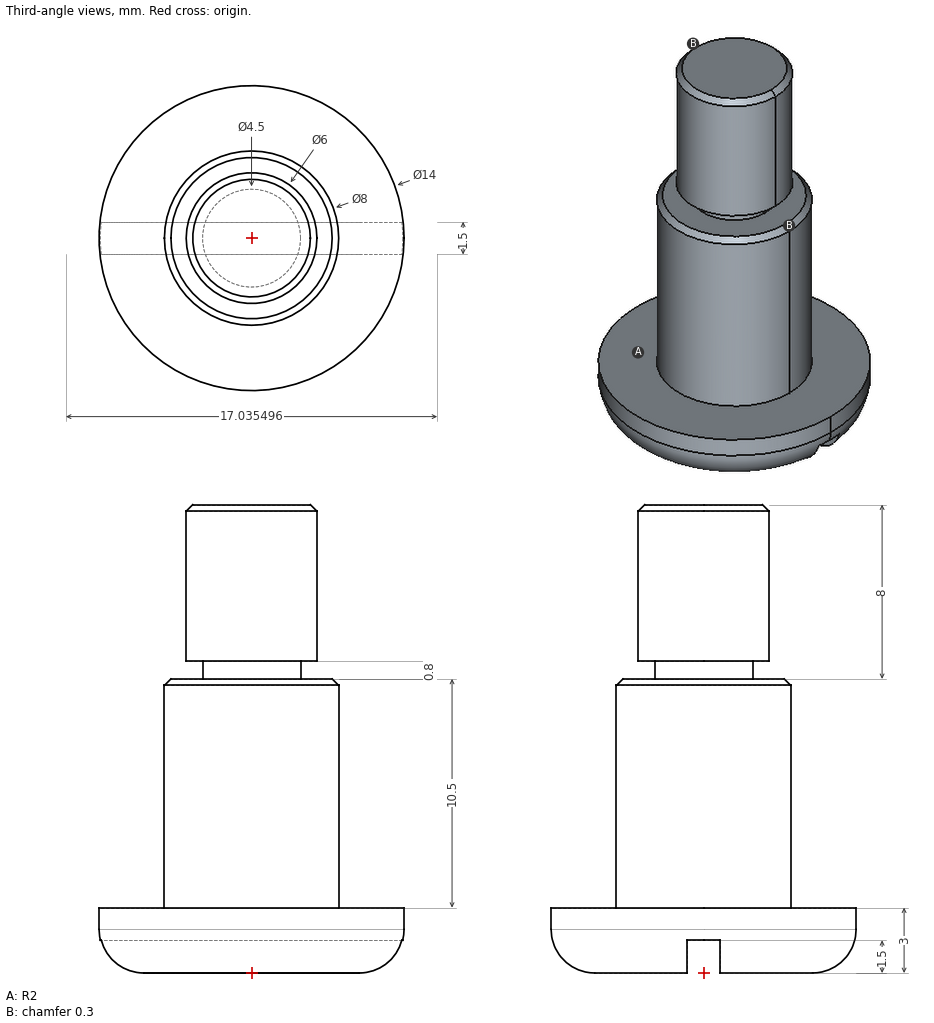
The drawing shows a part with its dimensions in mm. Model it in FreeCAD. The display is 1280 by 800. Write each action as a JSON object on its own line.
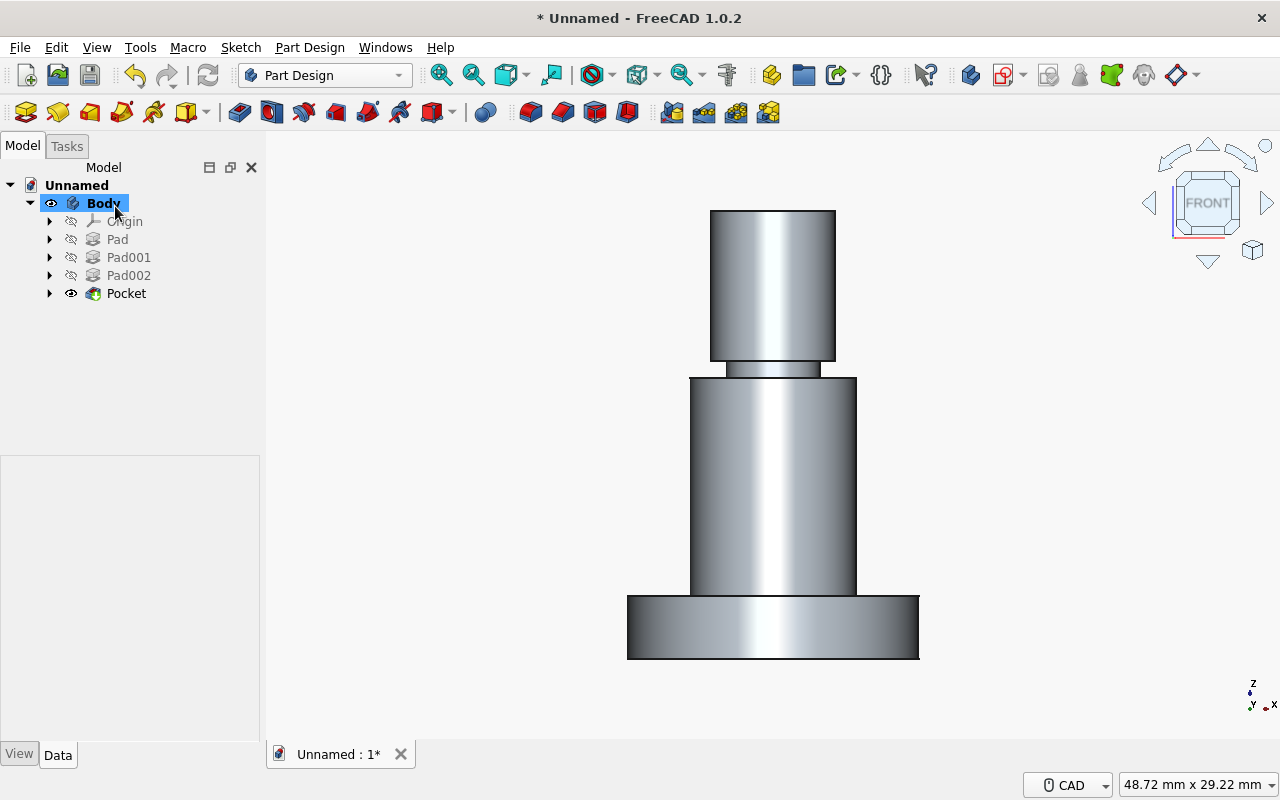
{"action": "left_click", "coordinate": [655, 658]}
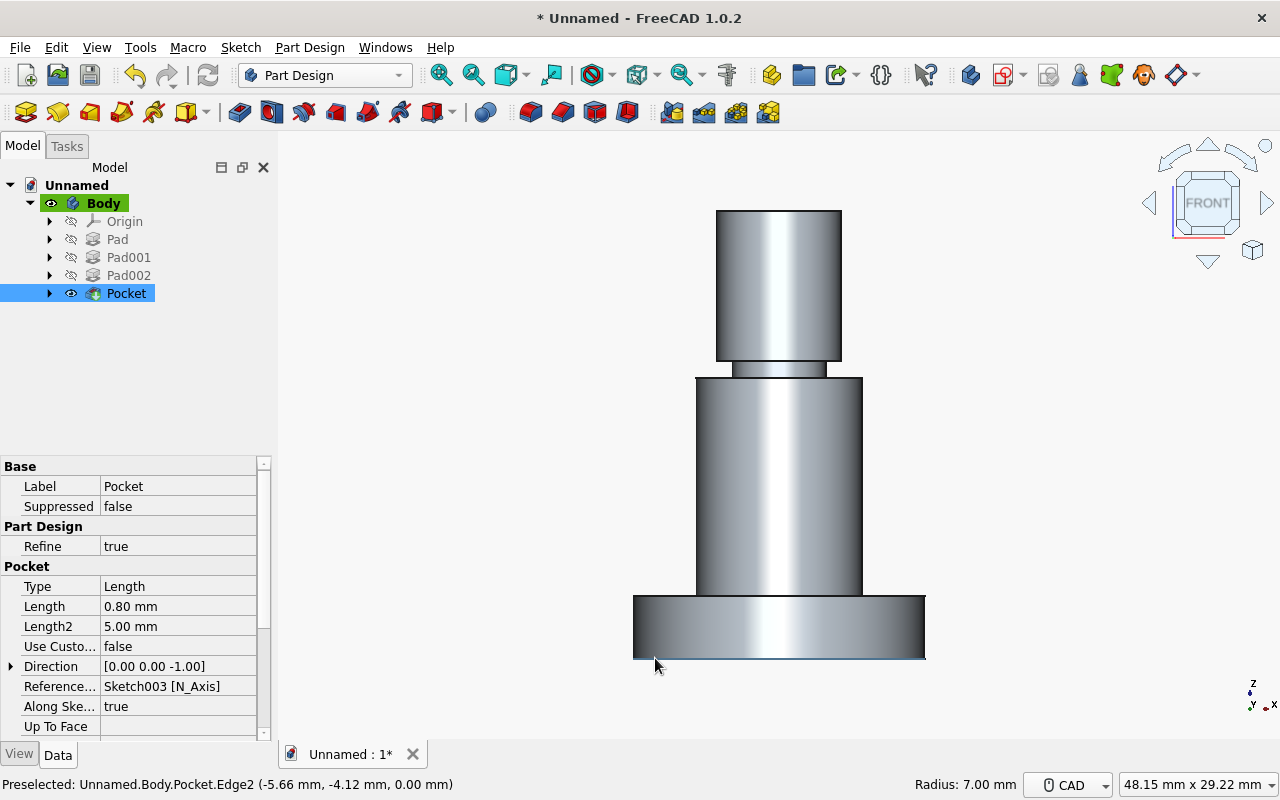
{"action": "left_click", "coordinate": [532, 112]}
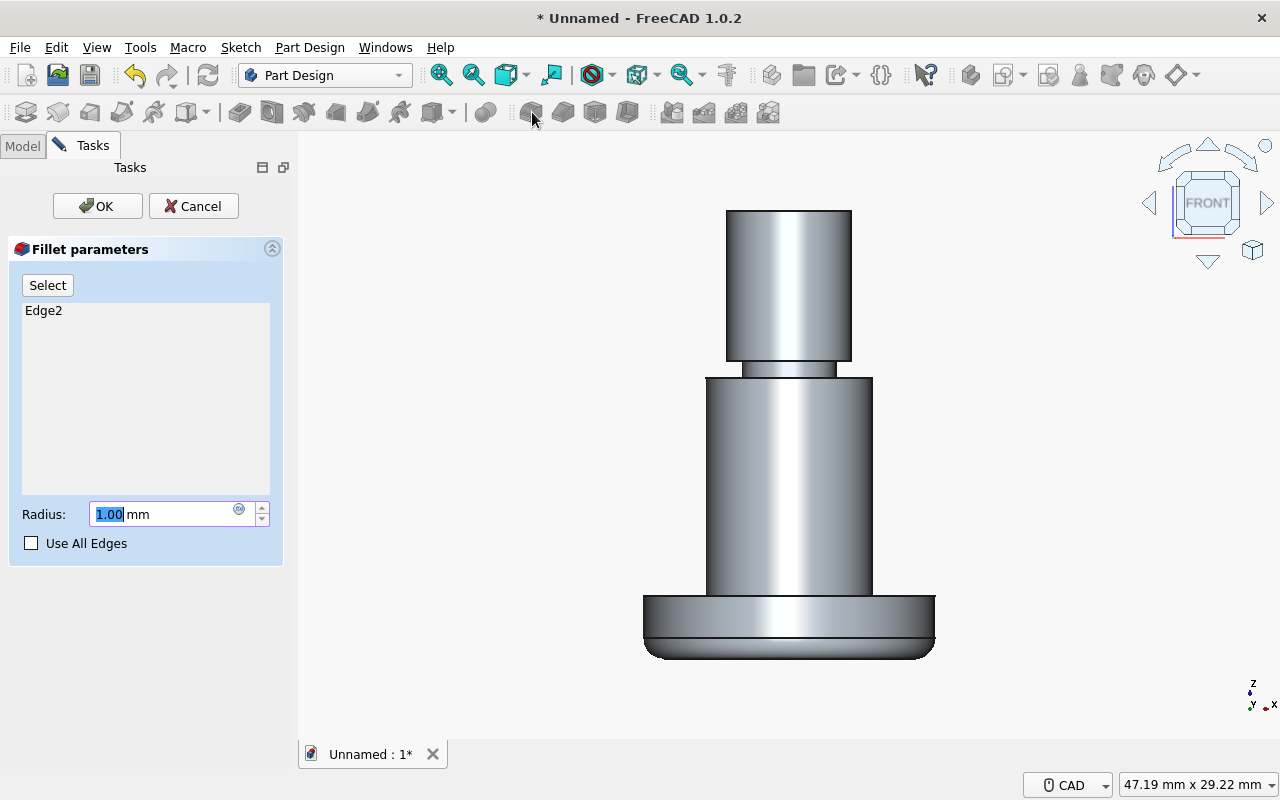
{"action": "type", "text": "2"}
{"action": "key", "text": "Tab"}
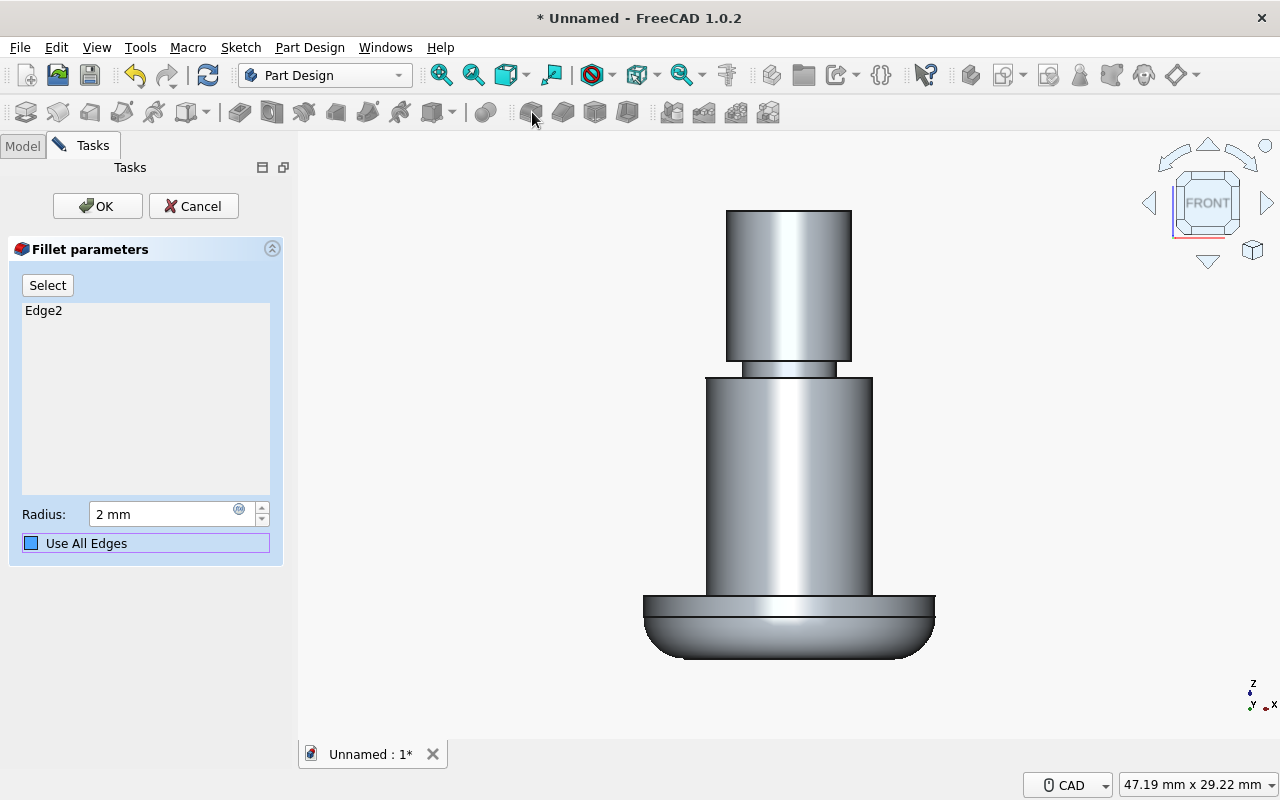
{"action": "left_click", "coordinate": [98, 206]}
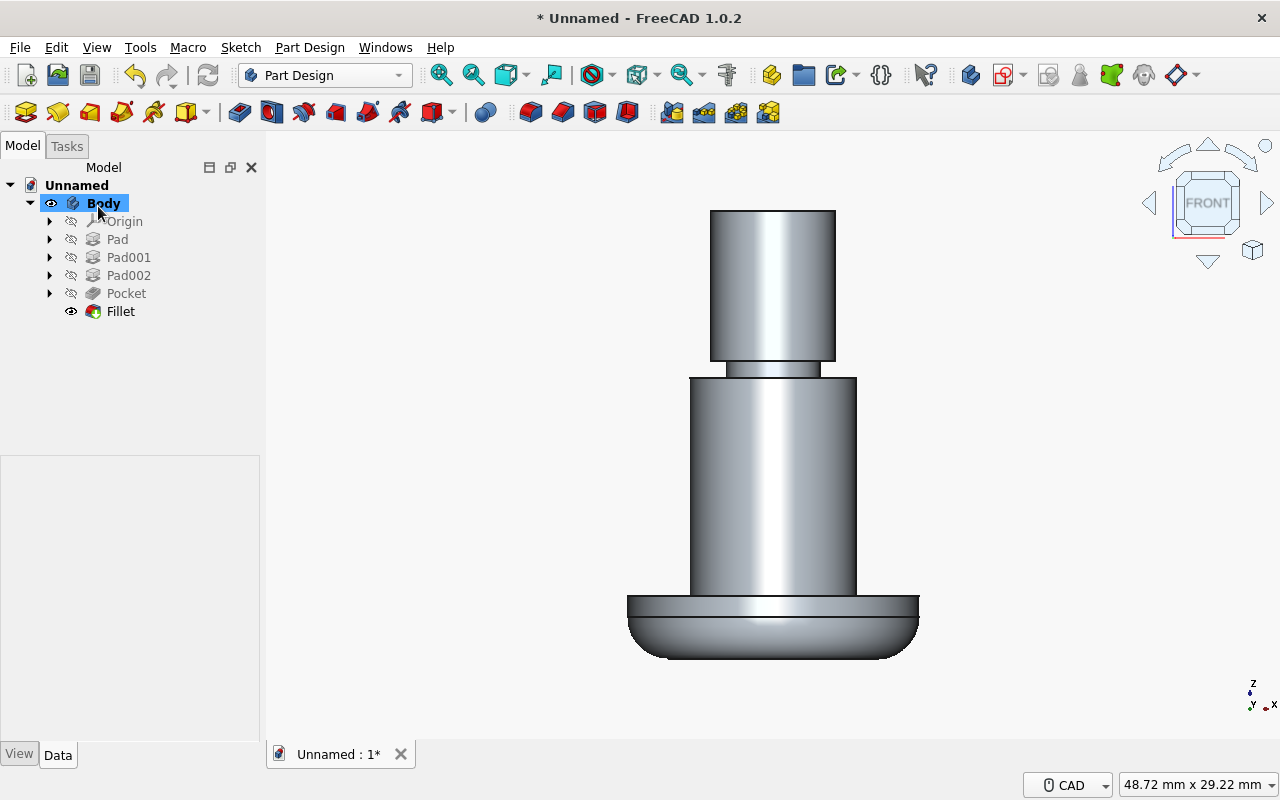
{"action": "left_click", "coordinate": [1004, 76]}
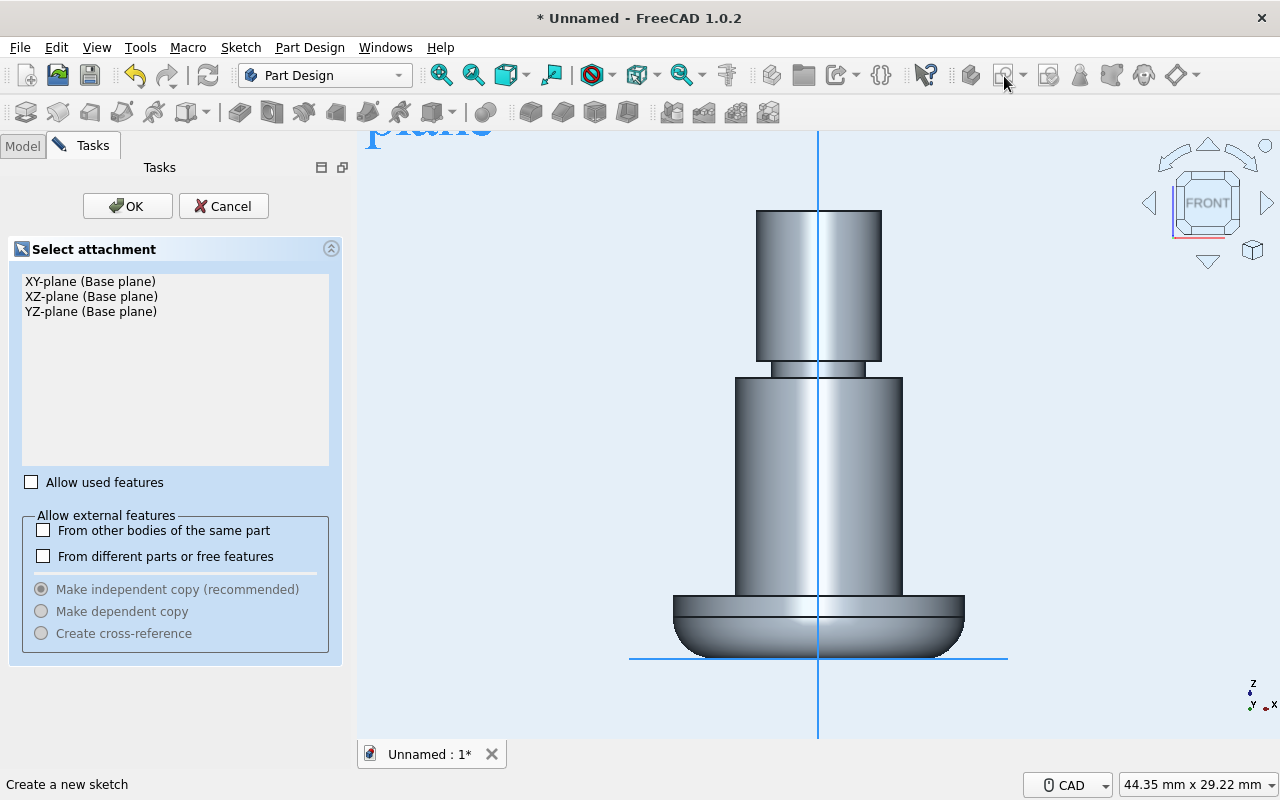
{"action": "left_click", "coordinate": [82, 282]}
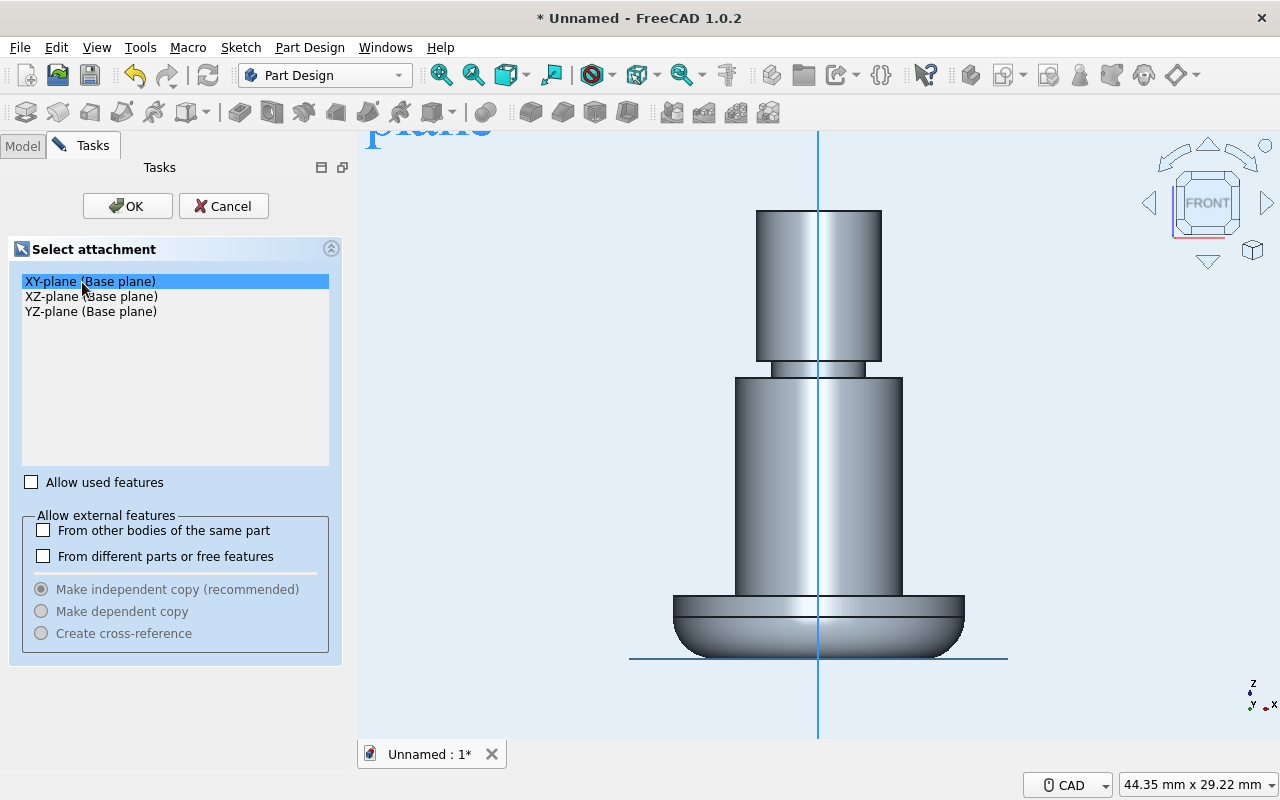
{"action": "left_click", "coordinate": [128, 206]}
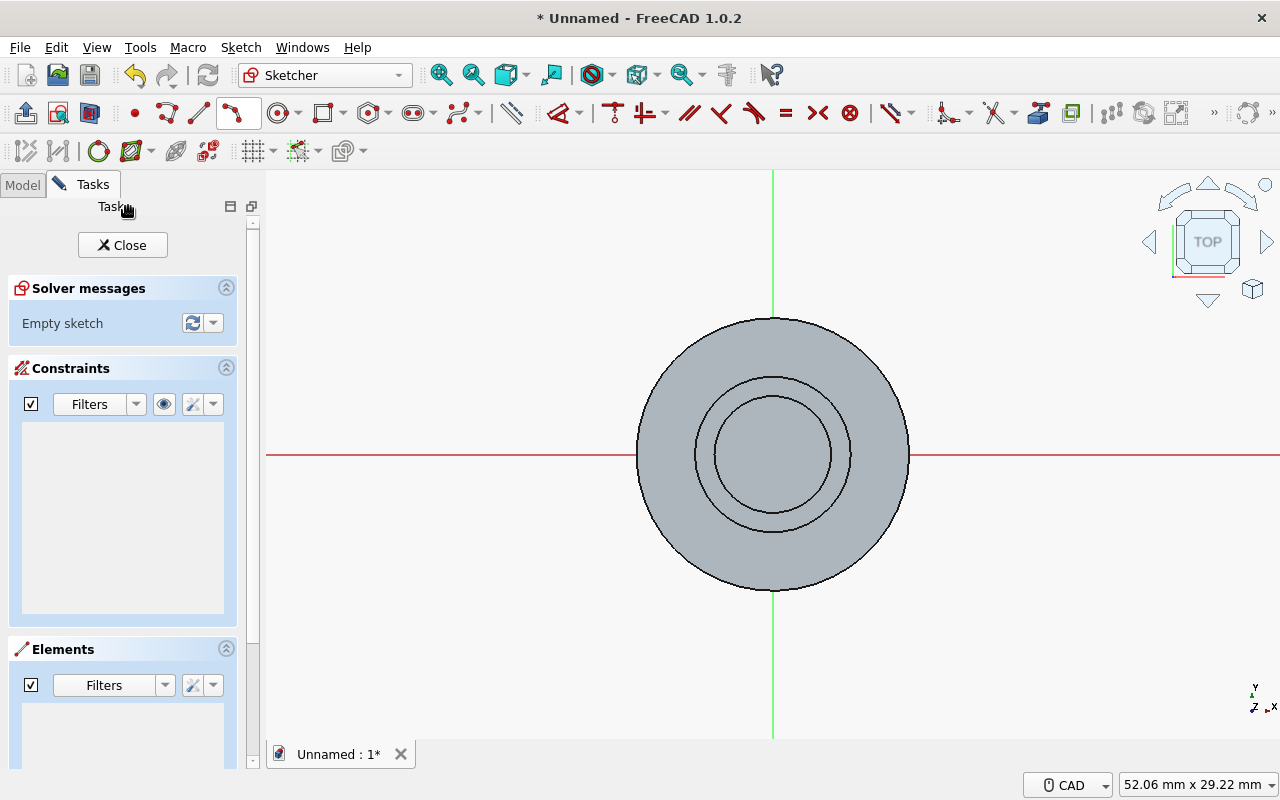
{"action": "left_click", "coordinate": [90, 114]}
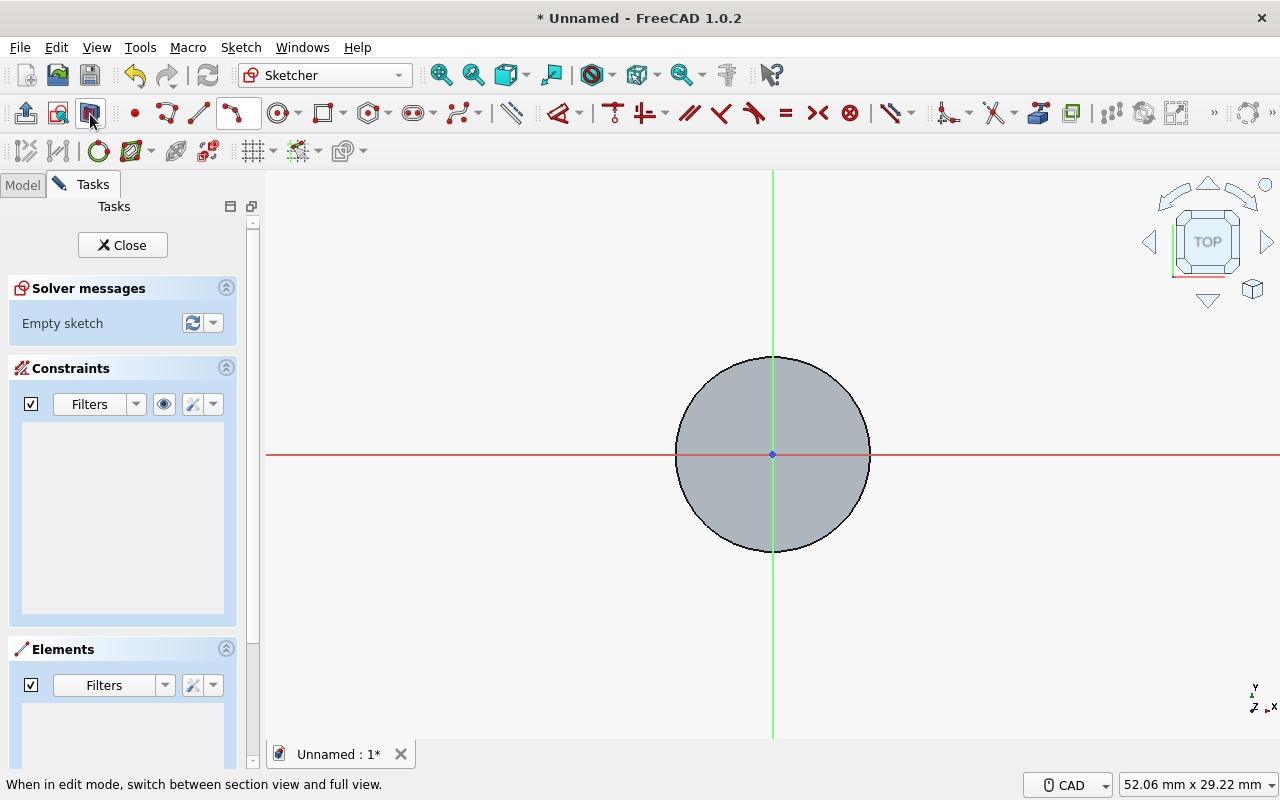
{"action": "scroll", "coordinate": [856, 454], "scroll_direction": "up", "scroll_amount": 3}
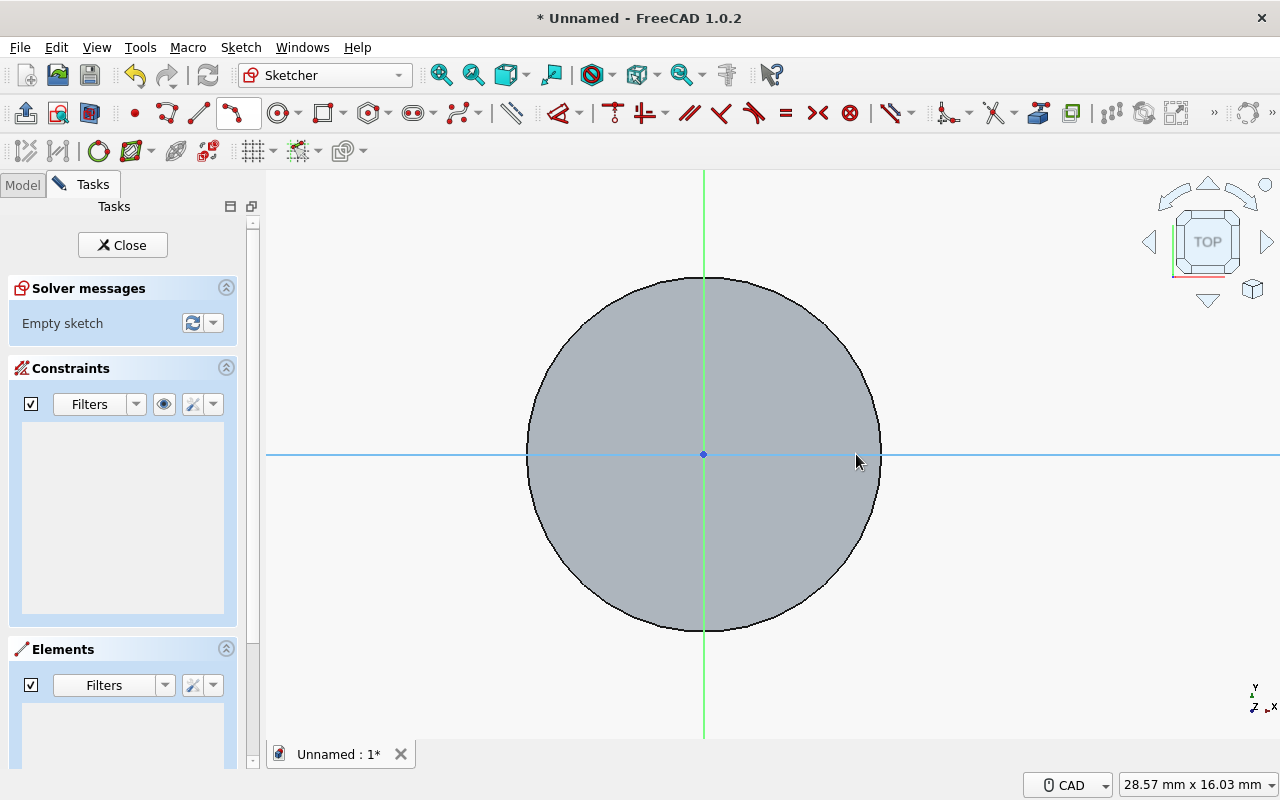
{"action": "left_click", "coordinate": [346, 114]}